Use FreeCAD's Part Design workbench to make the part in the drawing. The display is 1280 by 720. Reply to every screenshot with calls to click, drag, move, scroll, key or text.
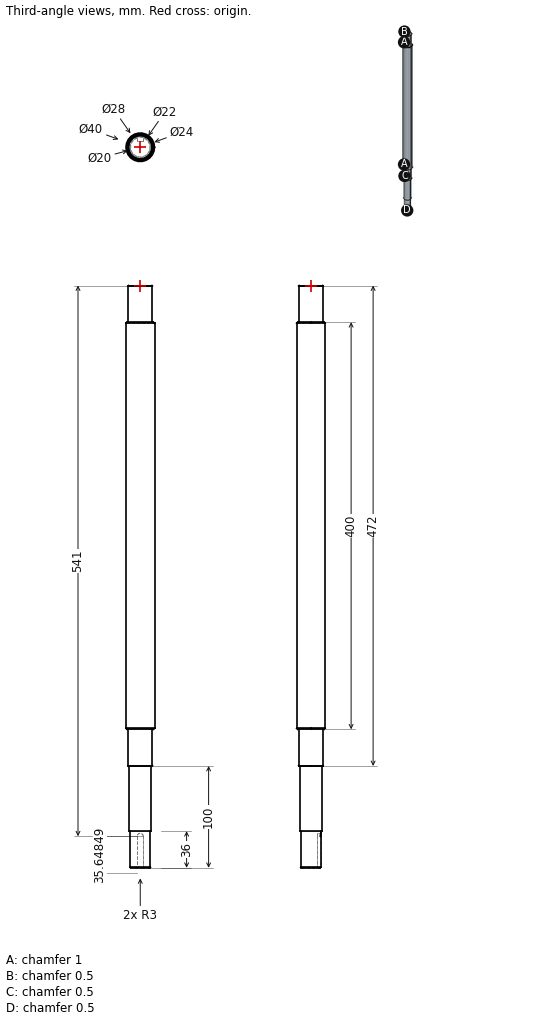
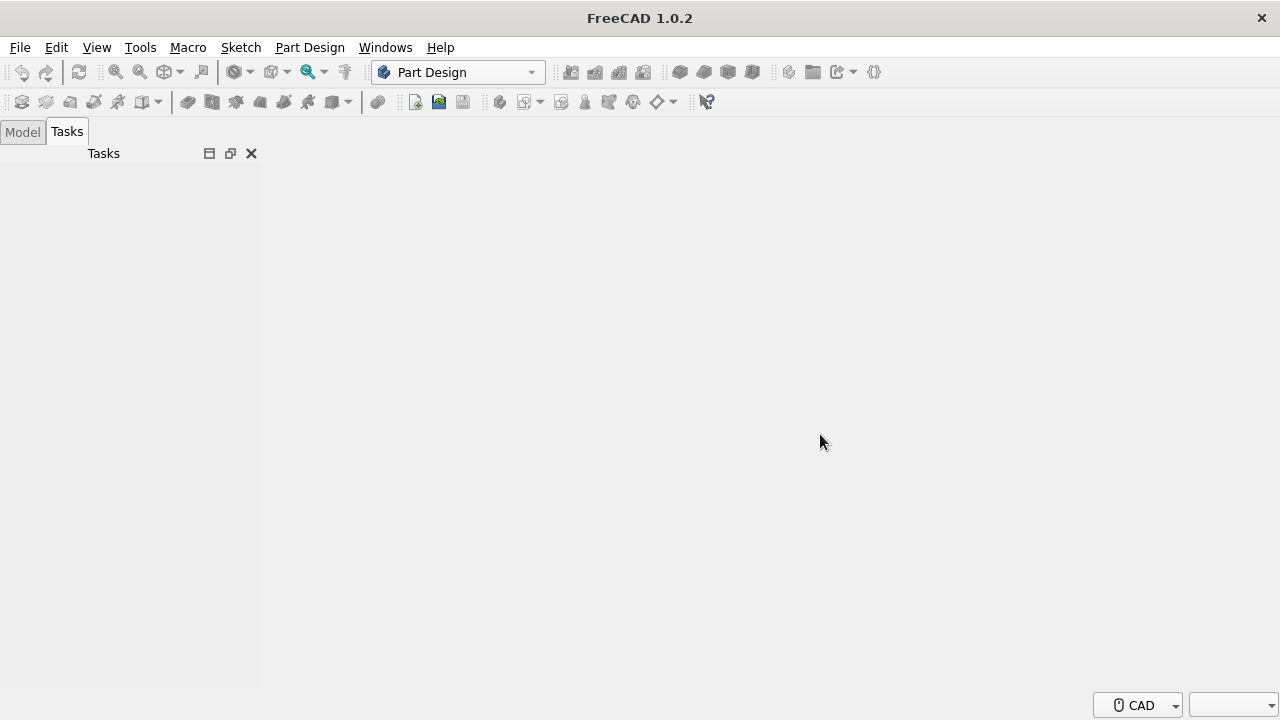
click(416, 102)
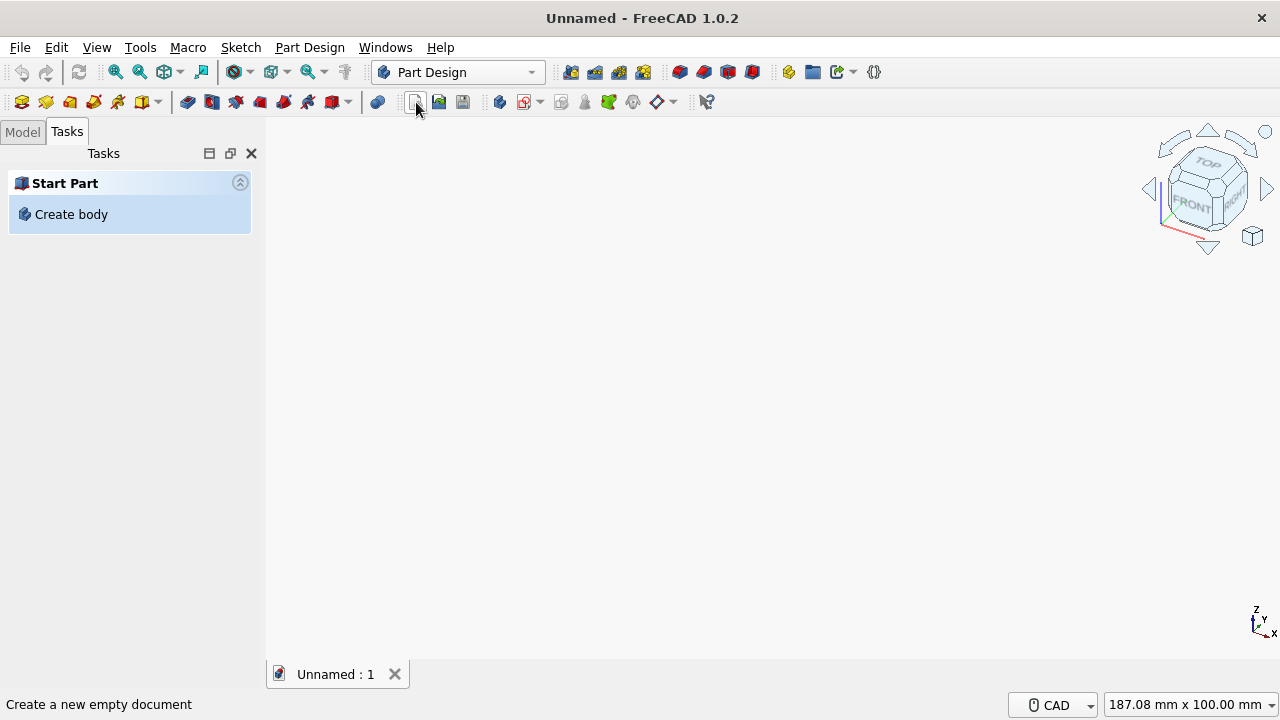
click(524, 102)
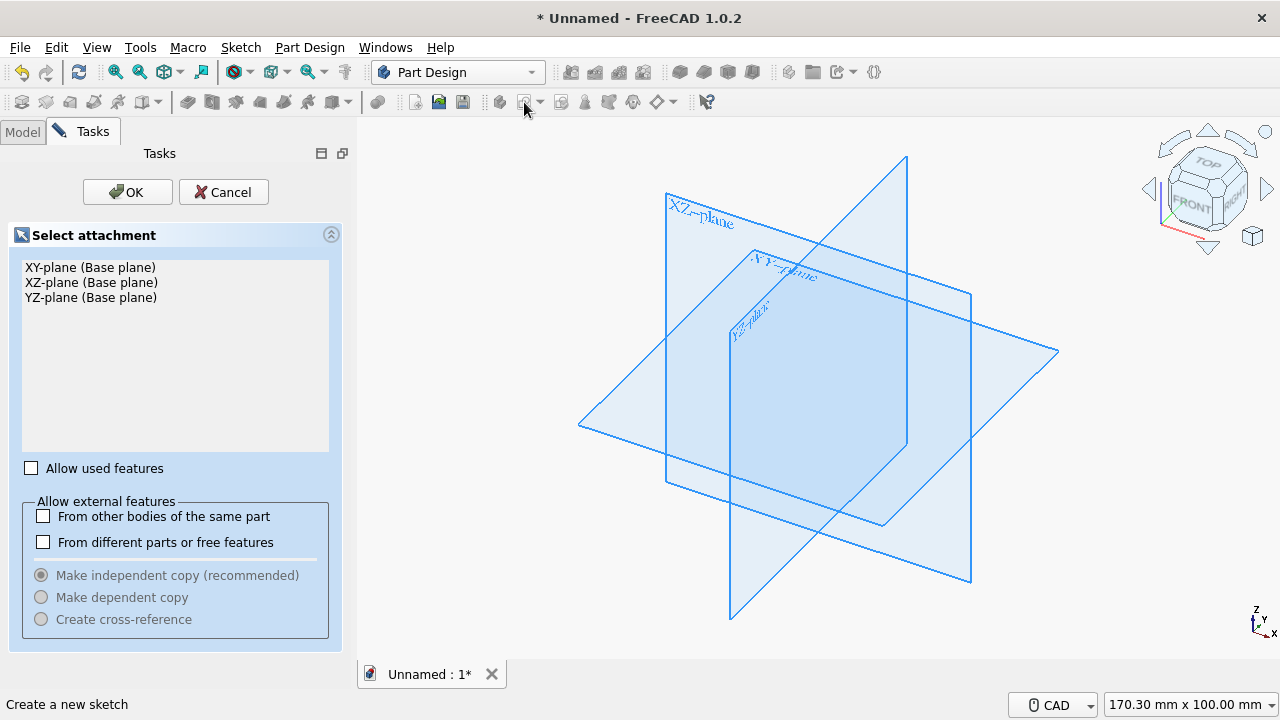
click(82, 268)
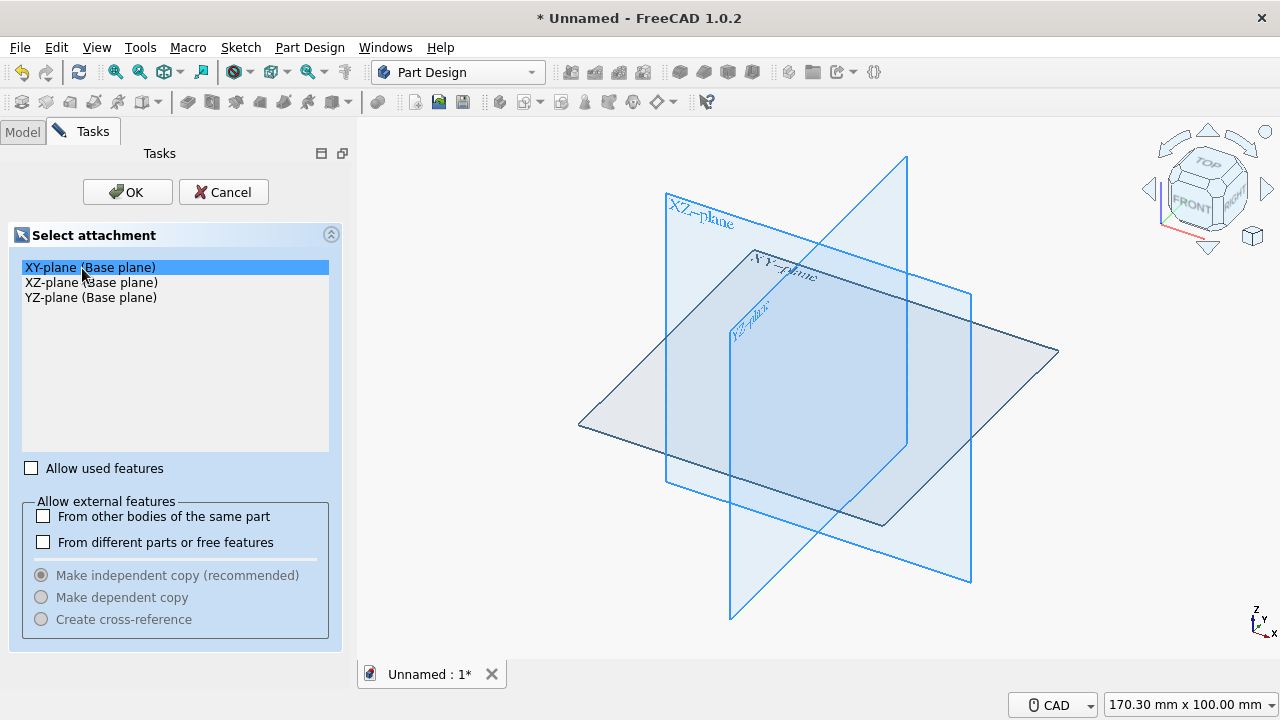
click(128, 192)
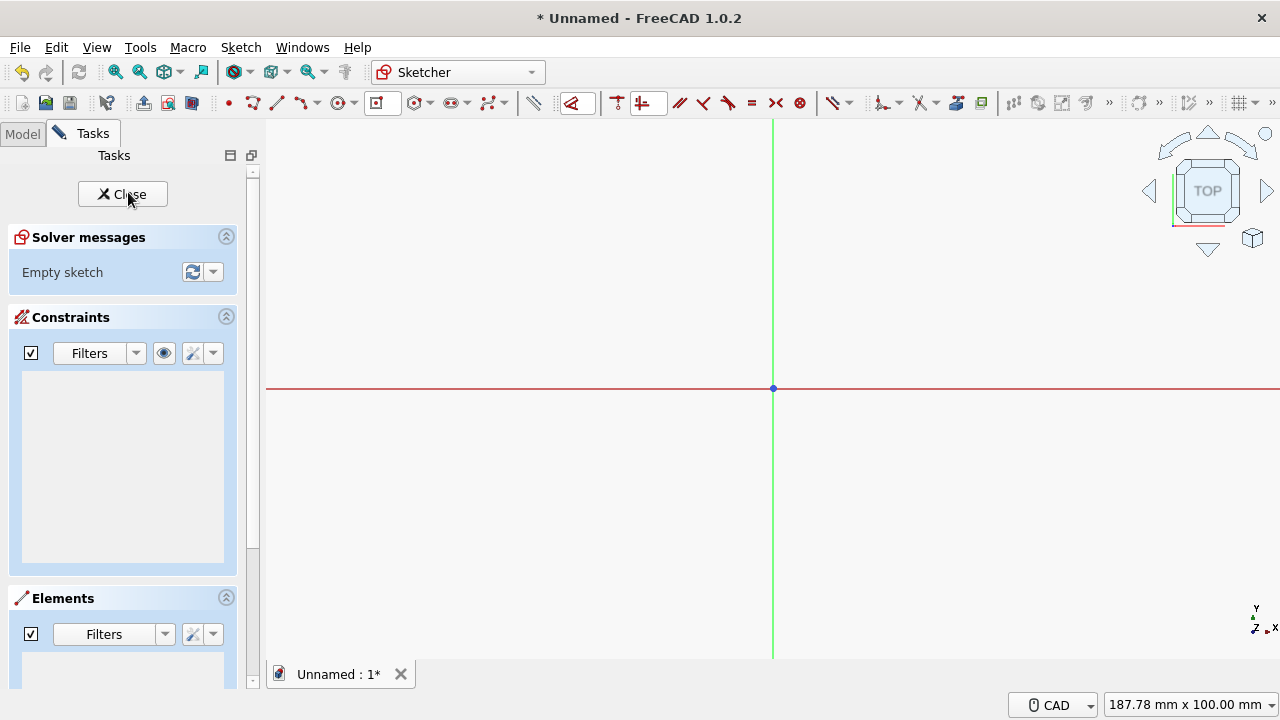
scroll(813, 389, up, 5)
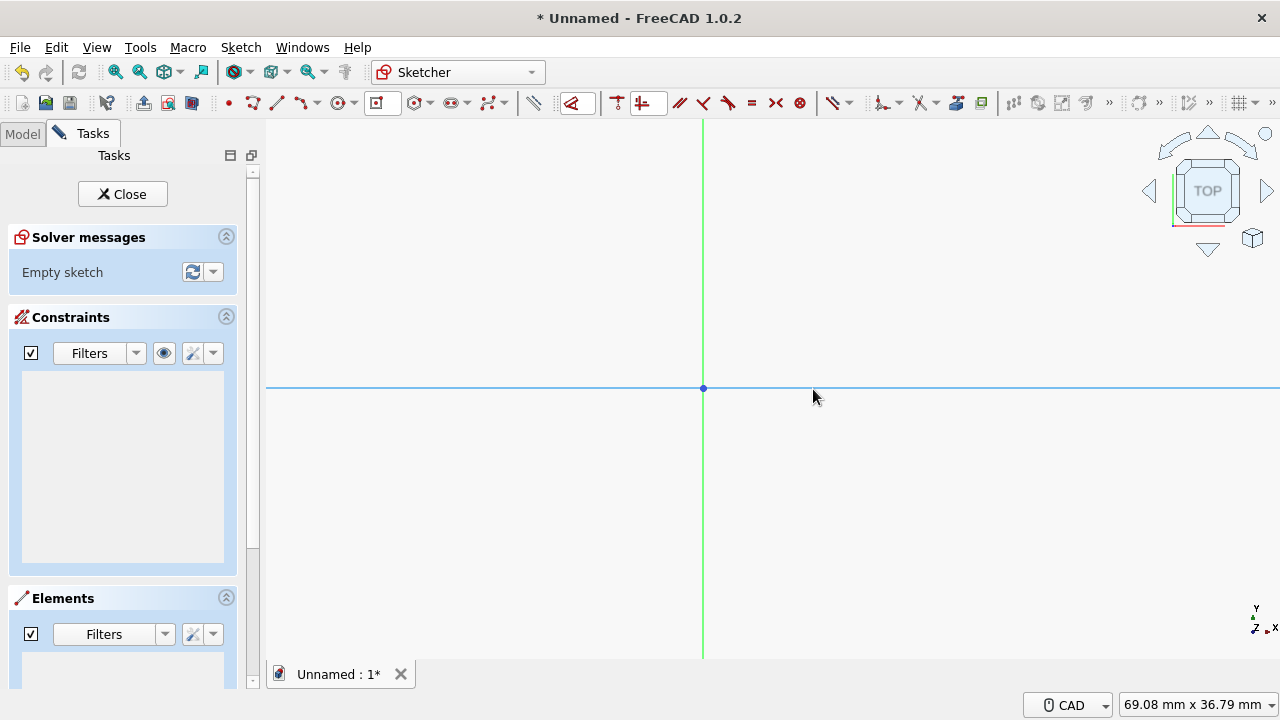
click(338, 104)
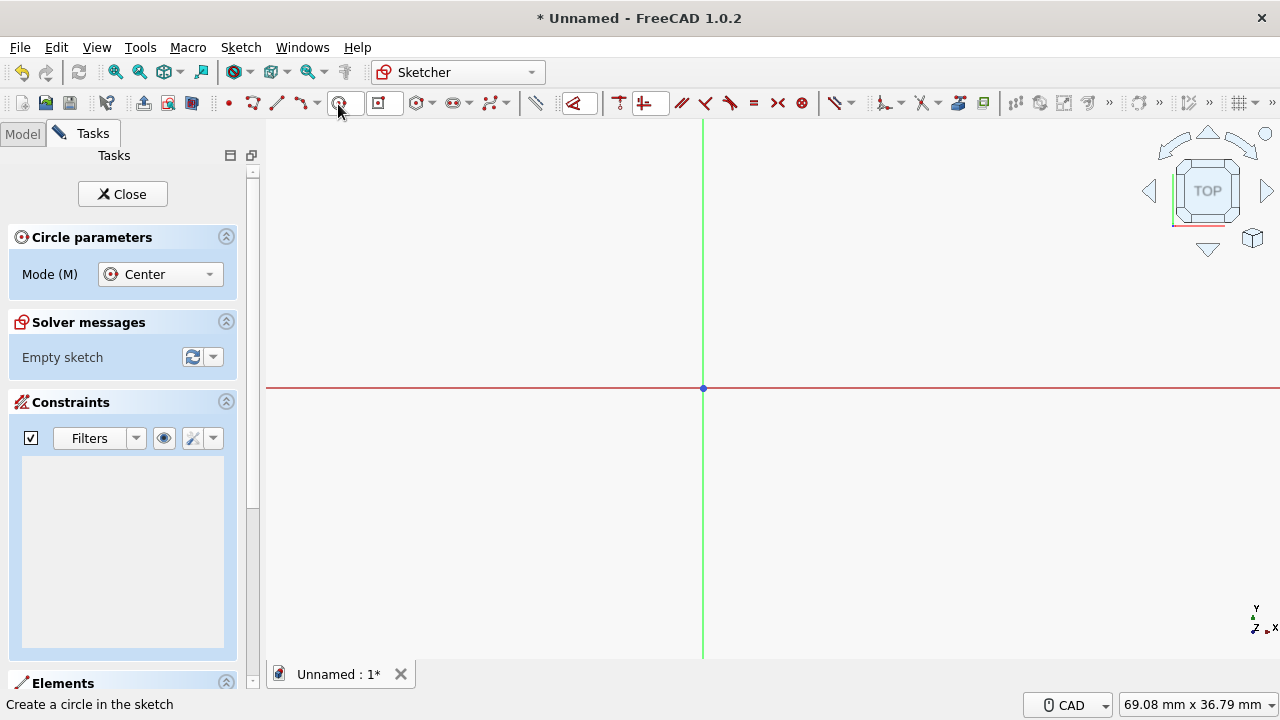
click(703, 388)
move(828, 264)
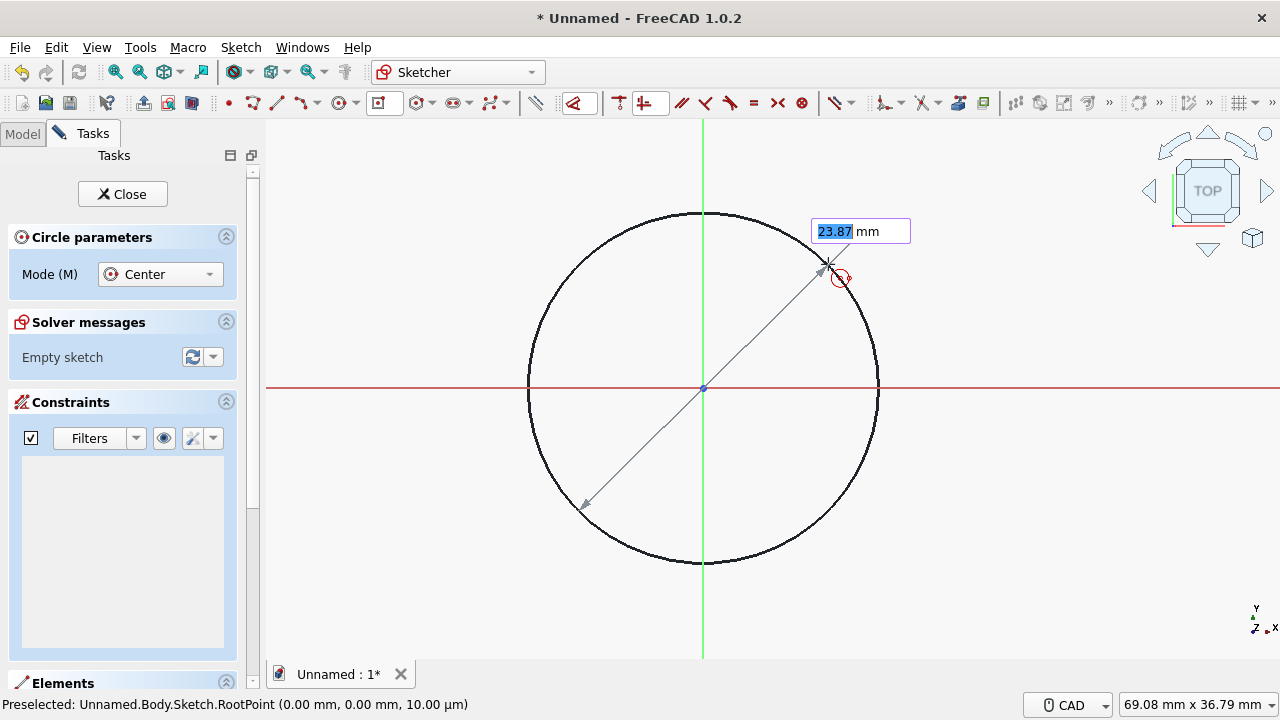
text(24)
key(Return)
key(Escape)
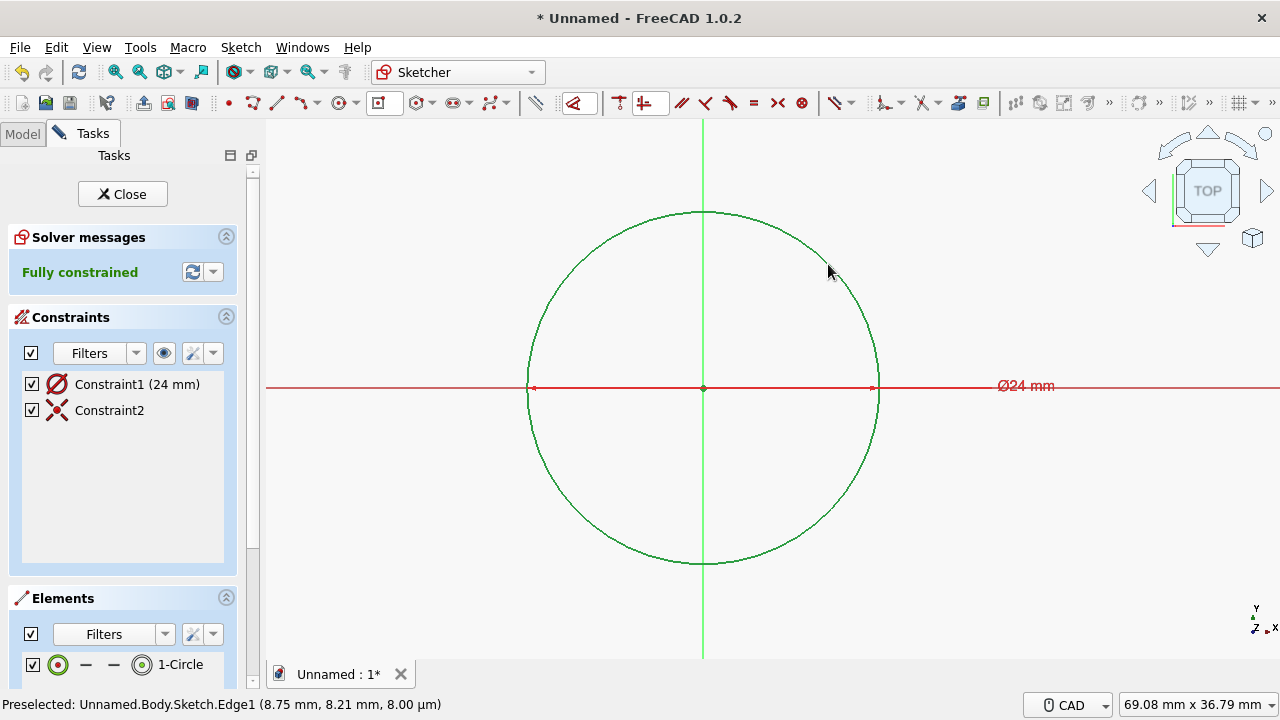
click(123, 194)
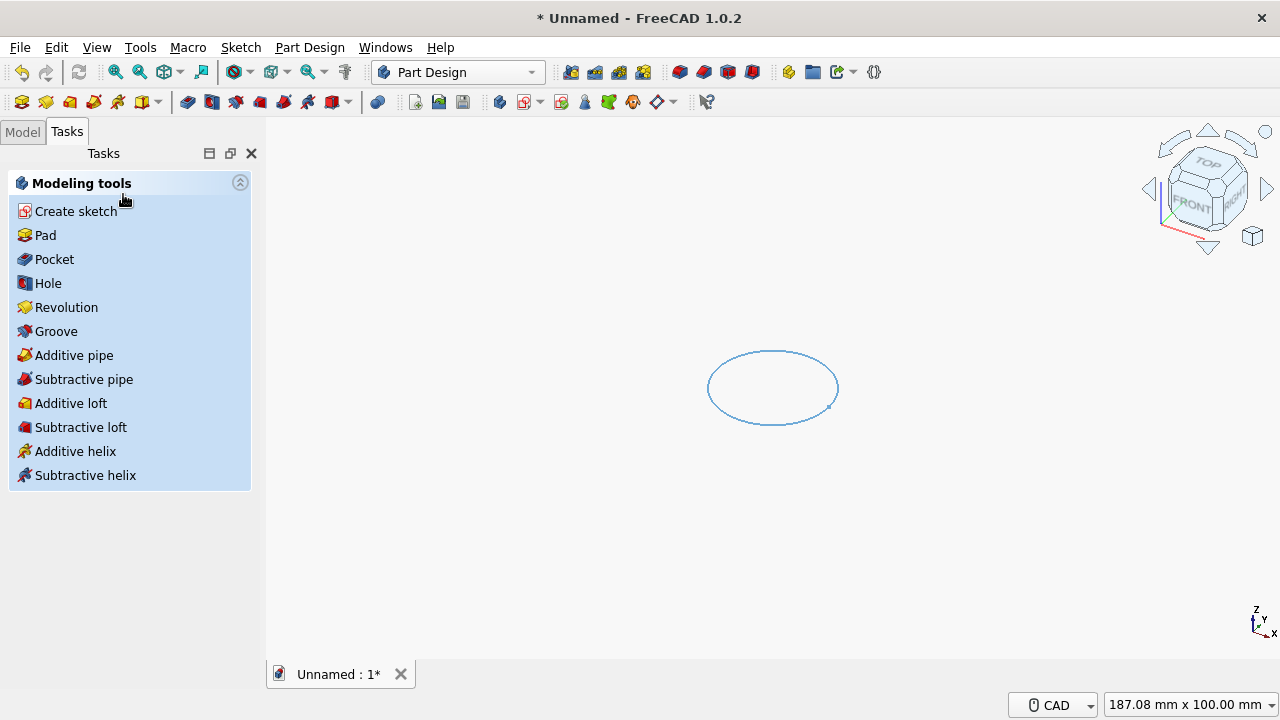
click(22, 102)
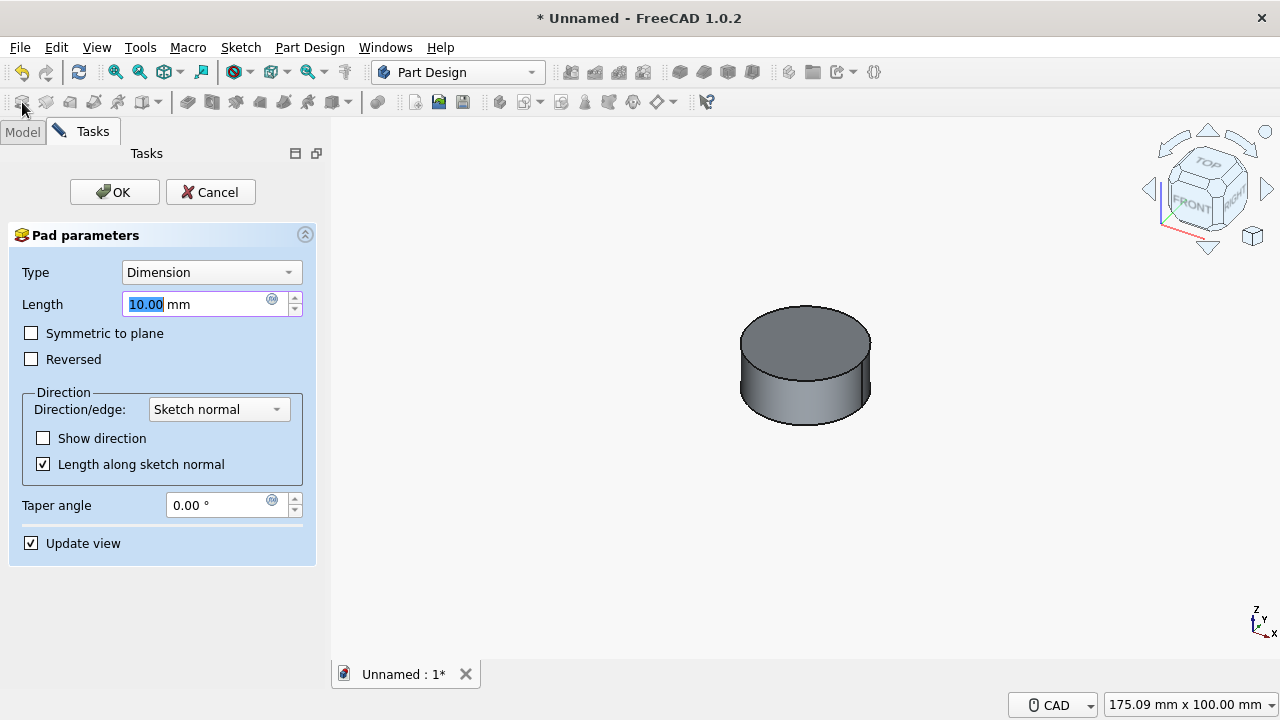
text(472)
key(Tab)